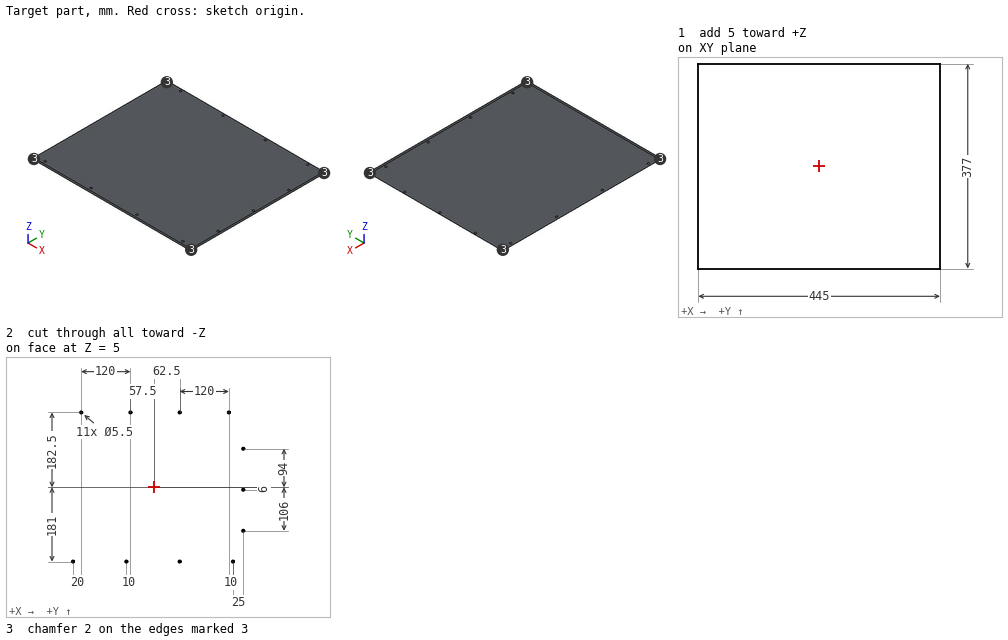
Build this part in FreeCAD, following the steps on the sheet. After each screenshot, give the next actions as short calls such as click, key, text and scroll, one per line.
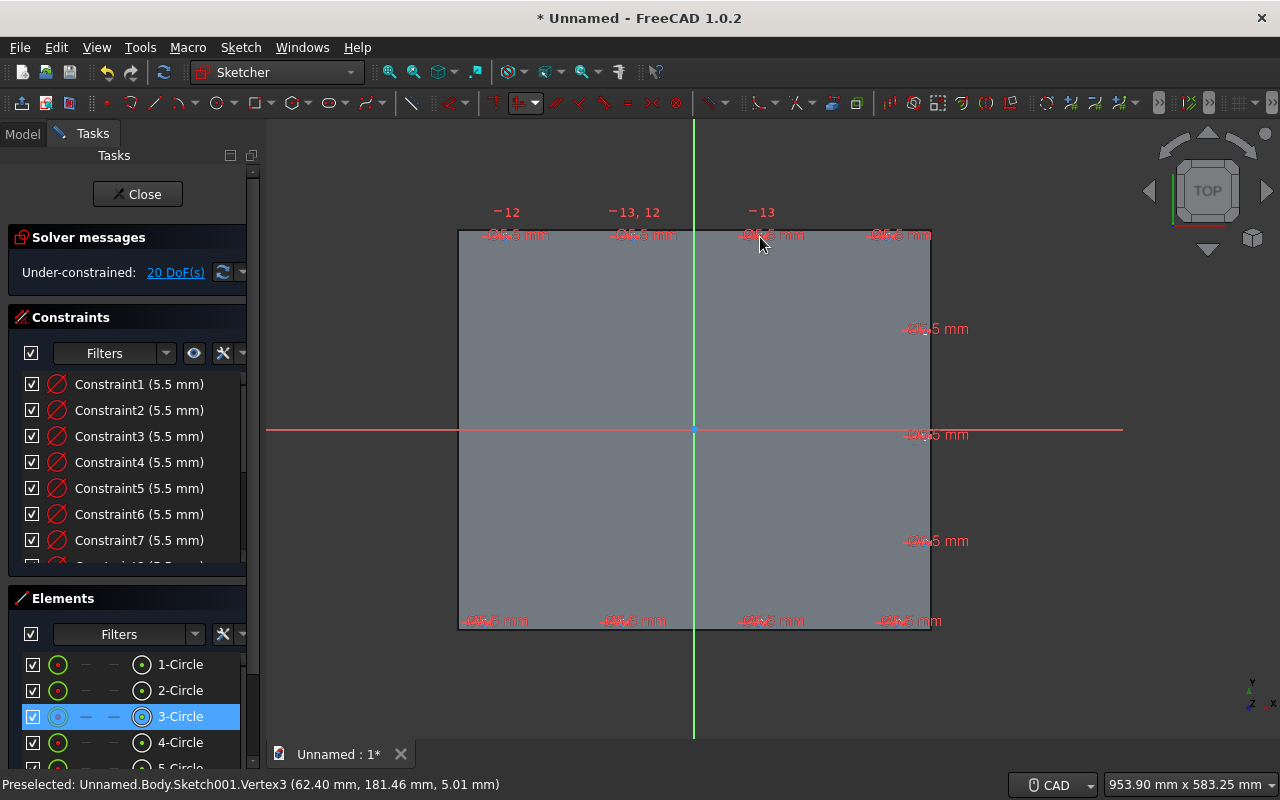
click(888, 237)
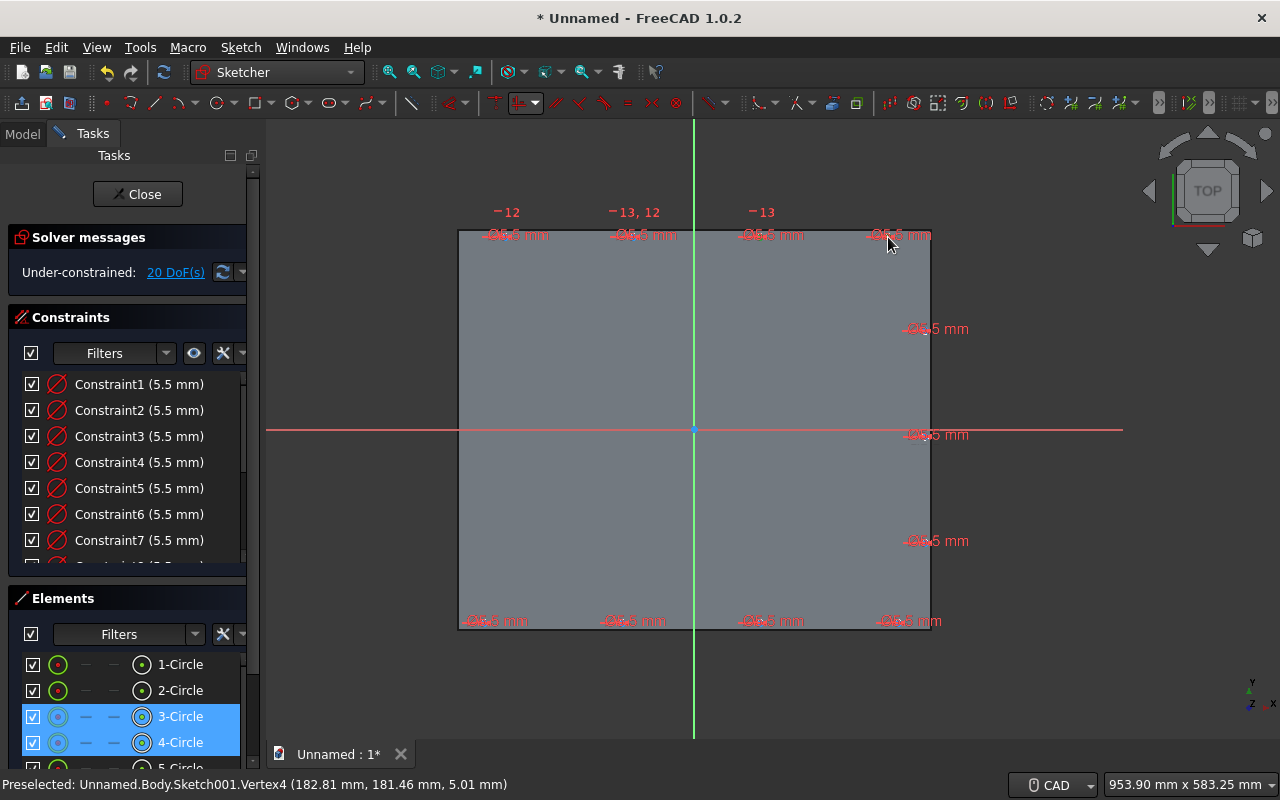
click(538, 104)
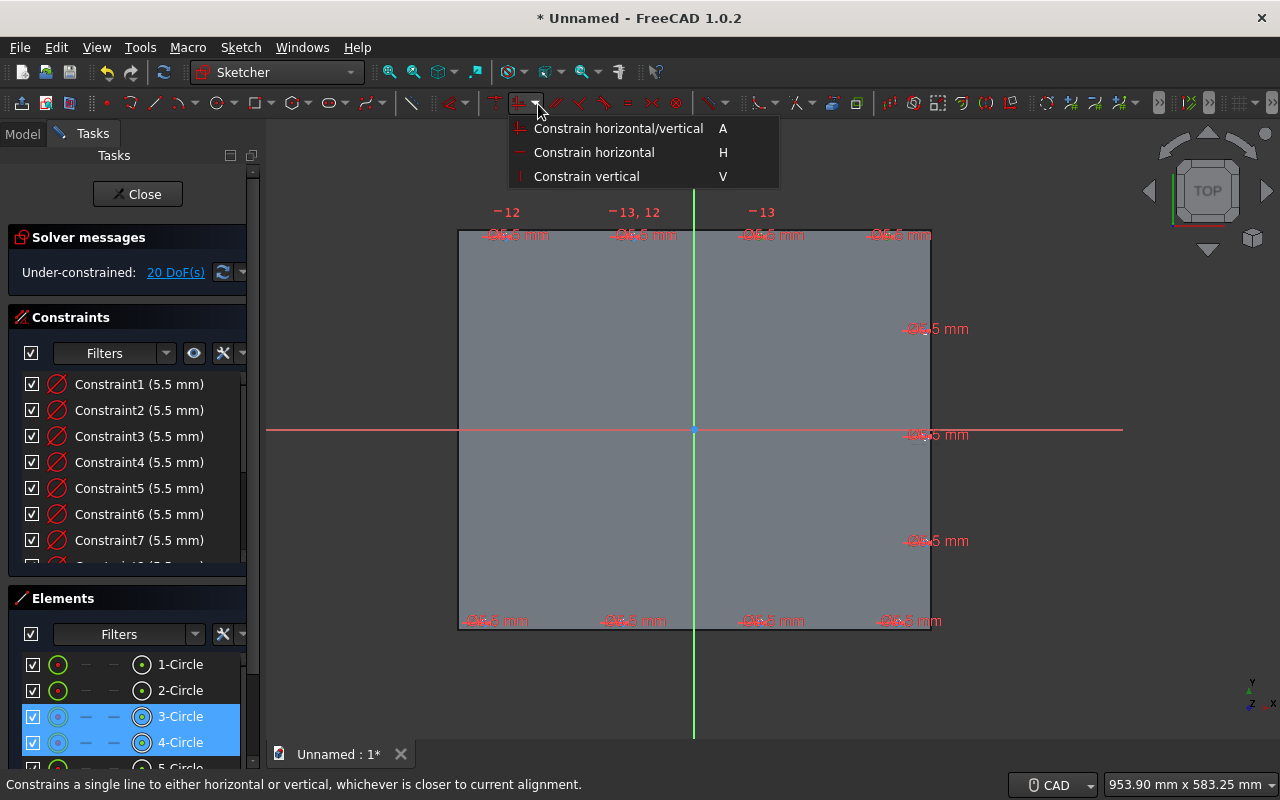
click(644, 152)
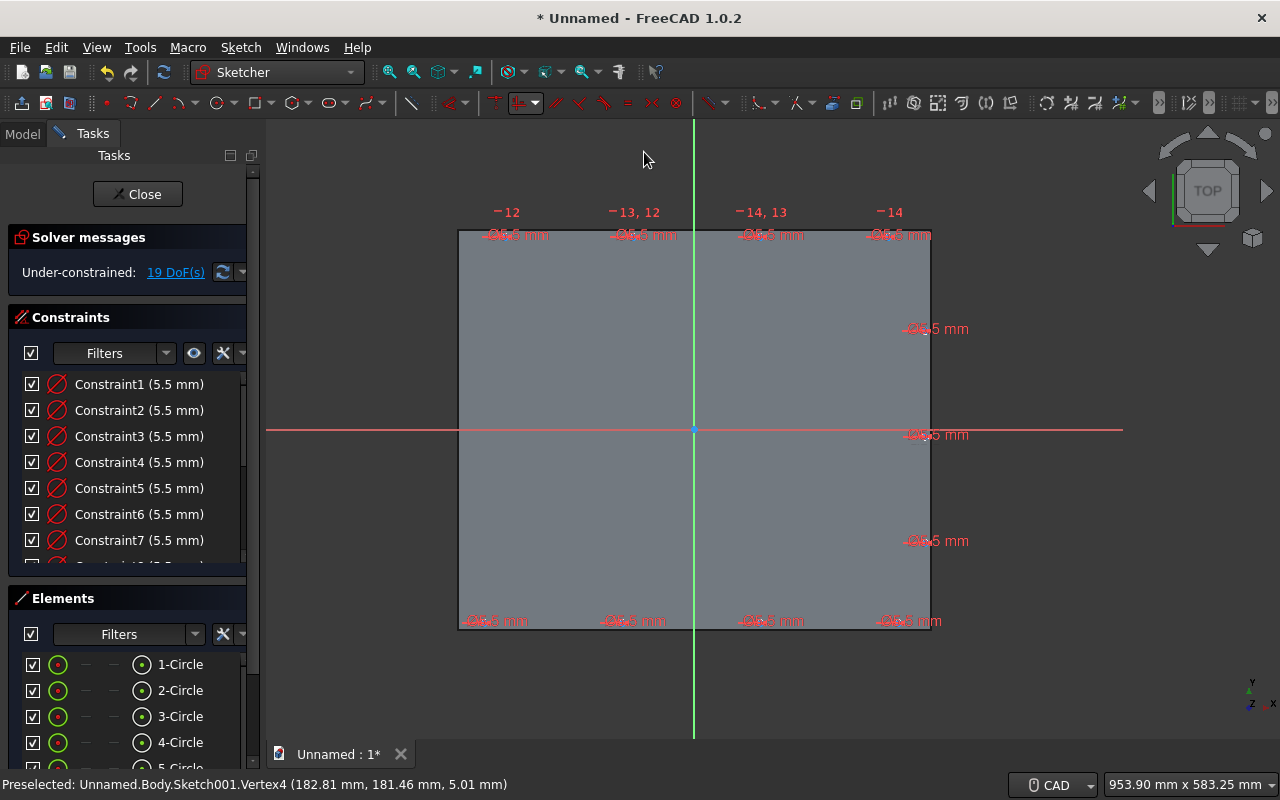
click(484, 623)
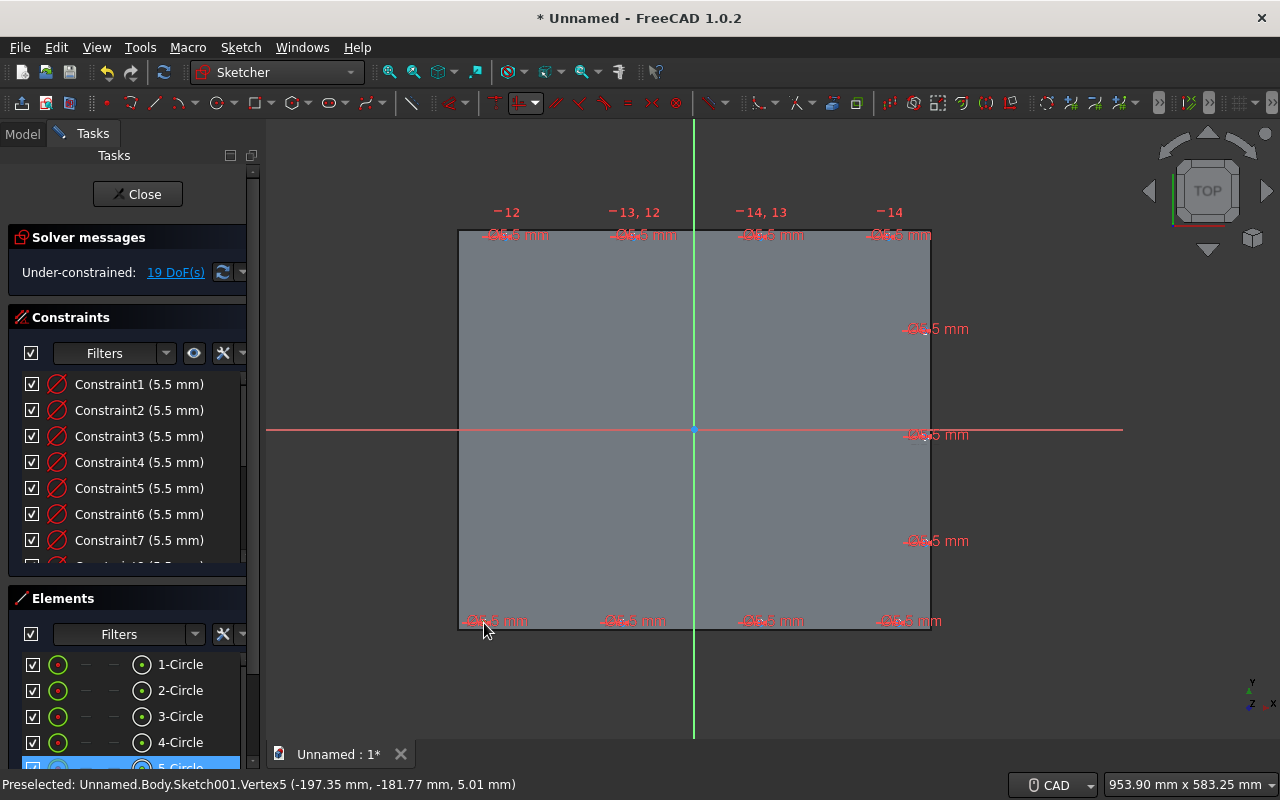
click(622, 623)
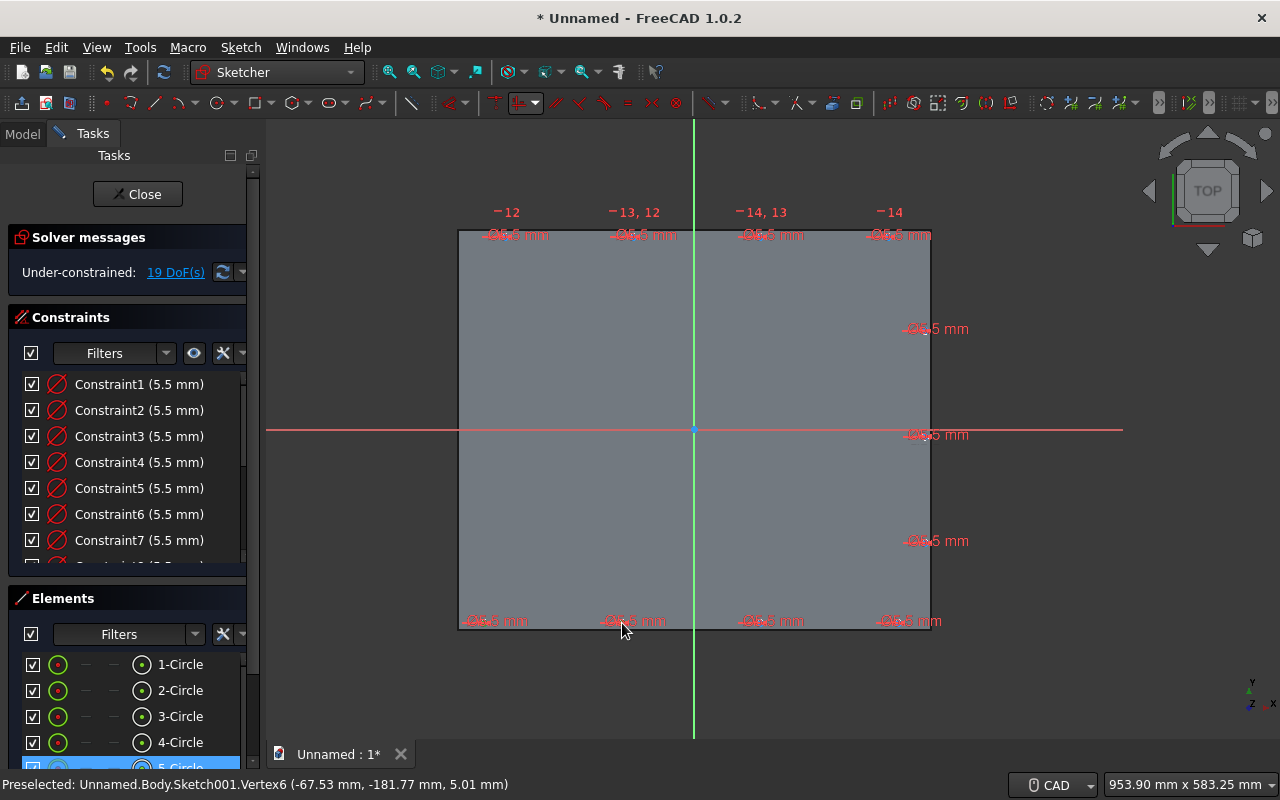
click(538, 104)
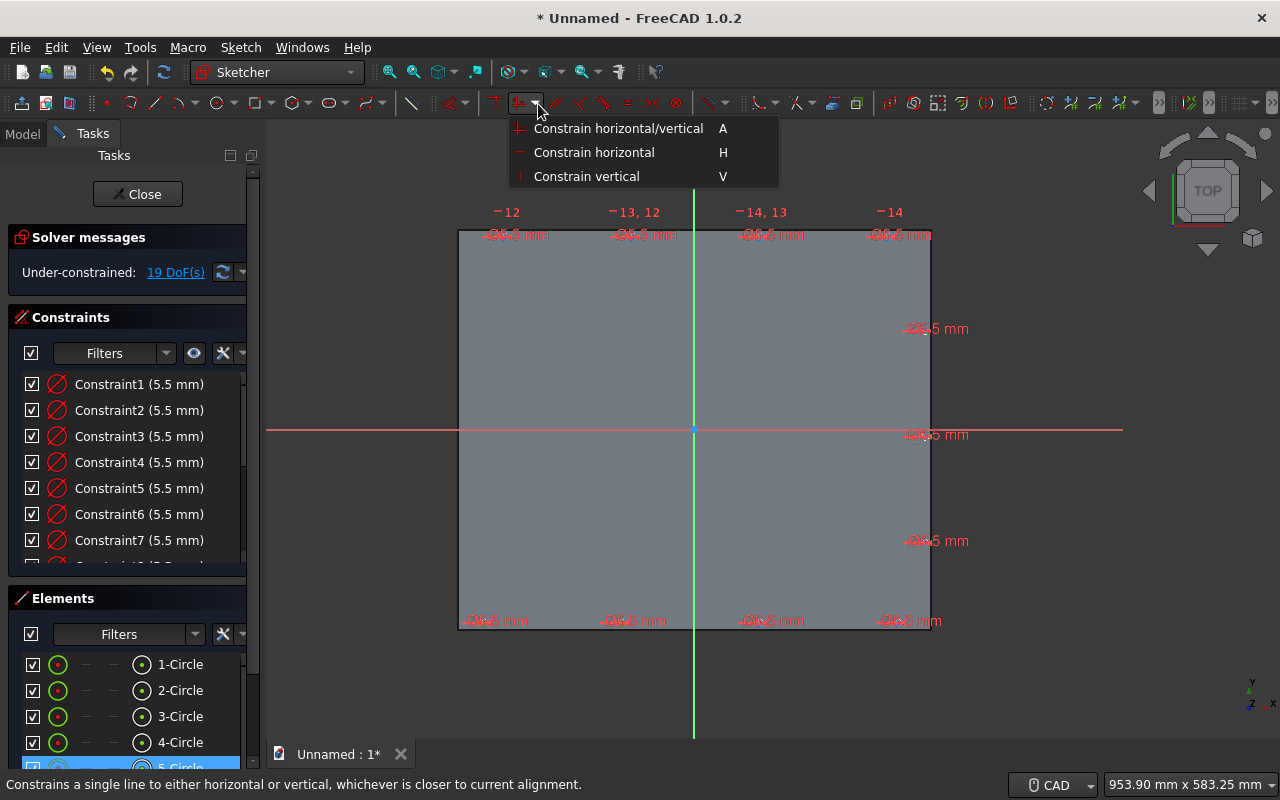
click(644, 152)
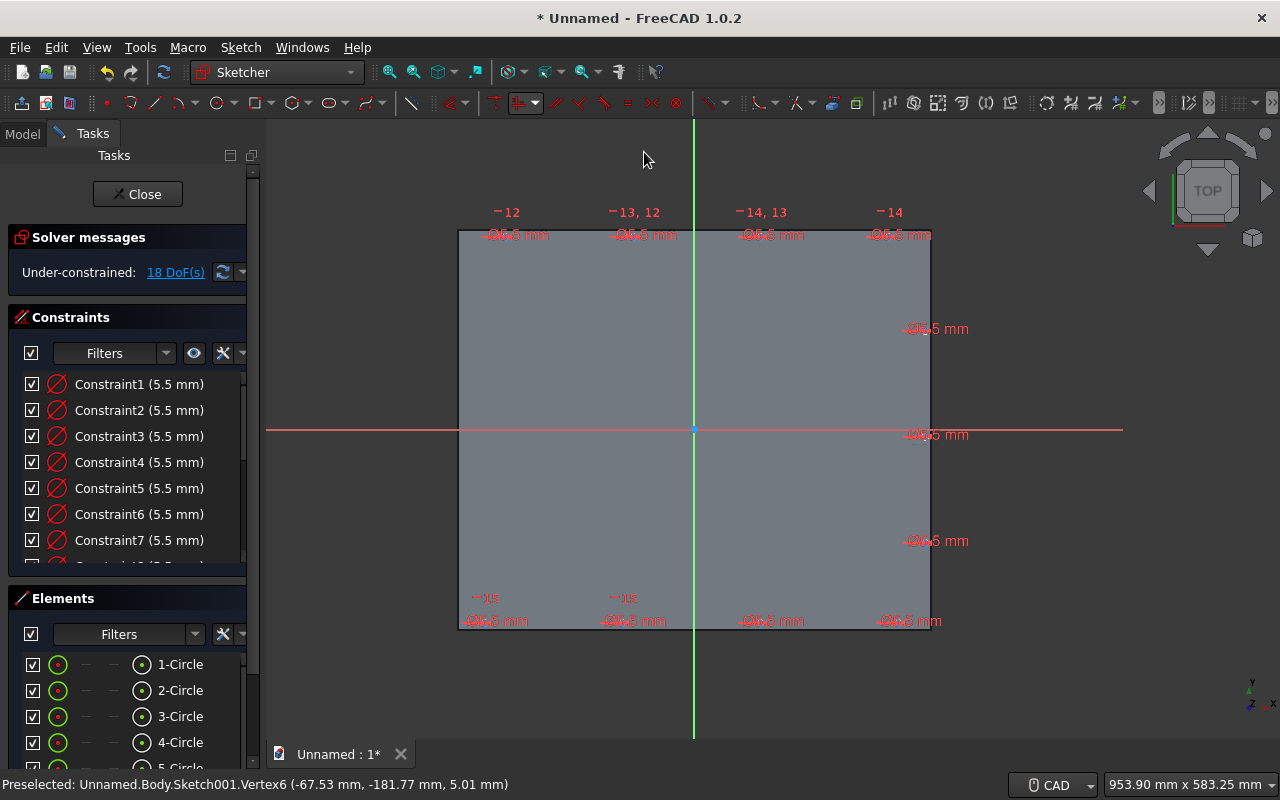
click(760, 237)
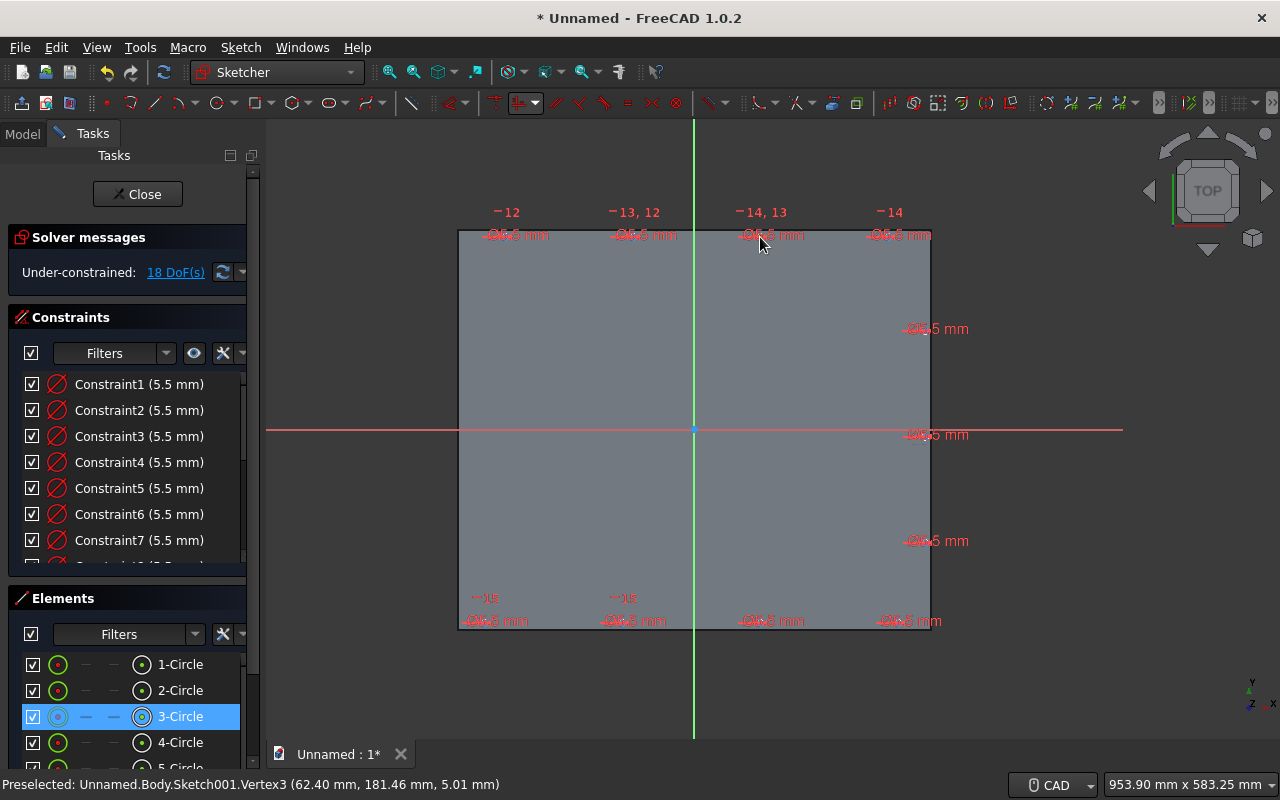
click(760, 623)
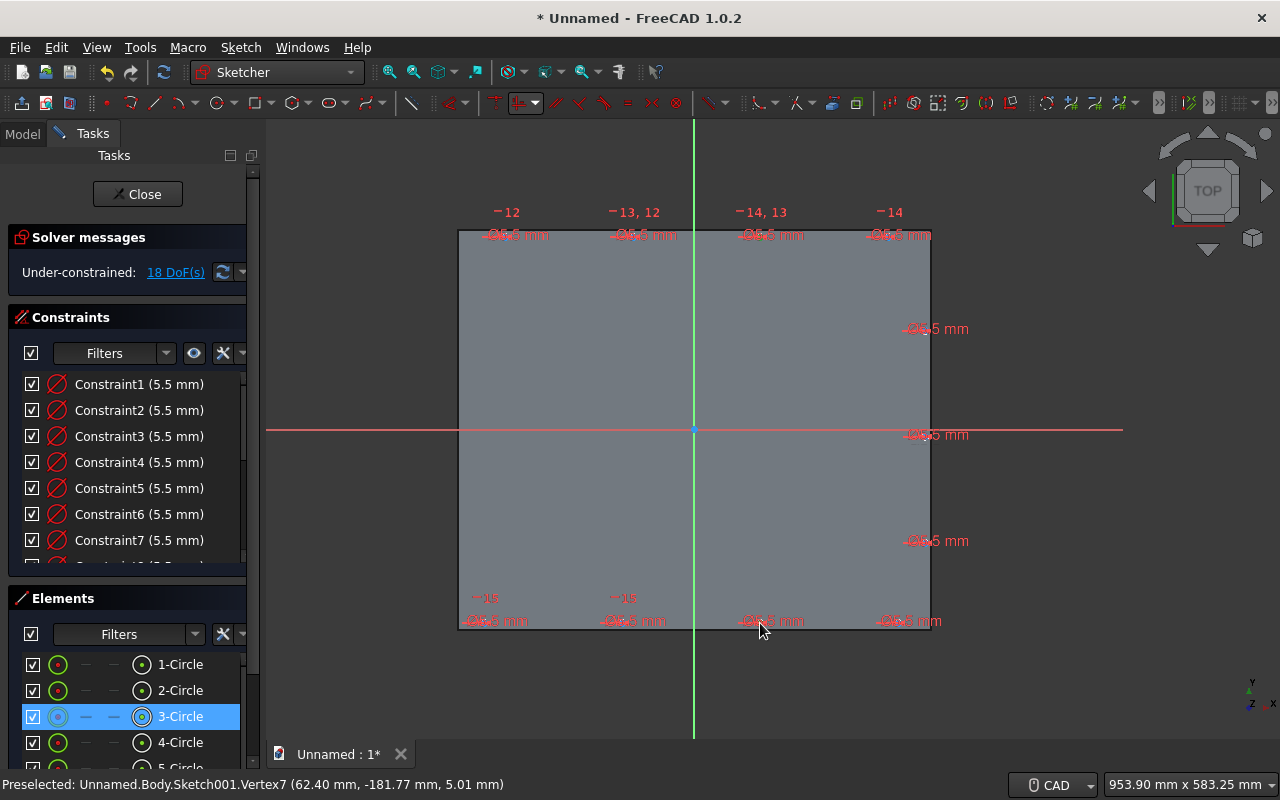
click(538, 104)